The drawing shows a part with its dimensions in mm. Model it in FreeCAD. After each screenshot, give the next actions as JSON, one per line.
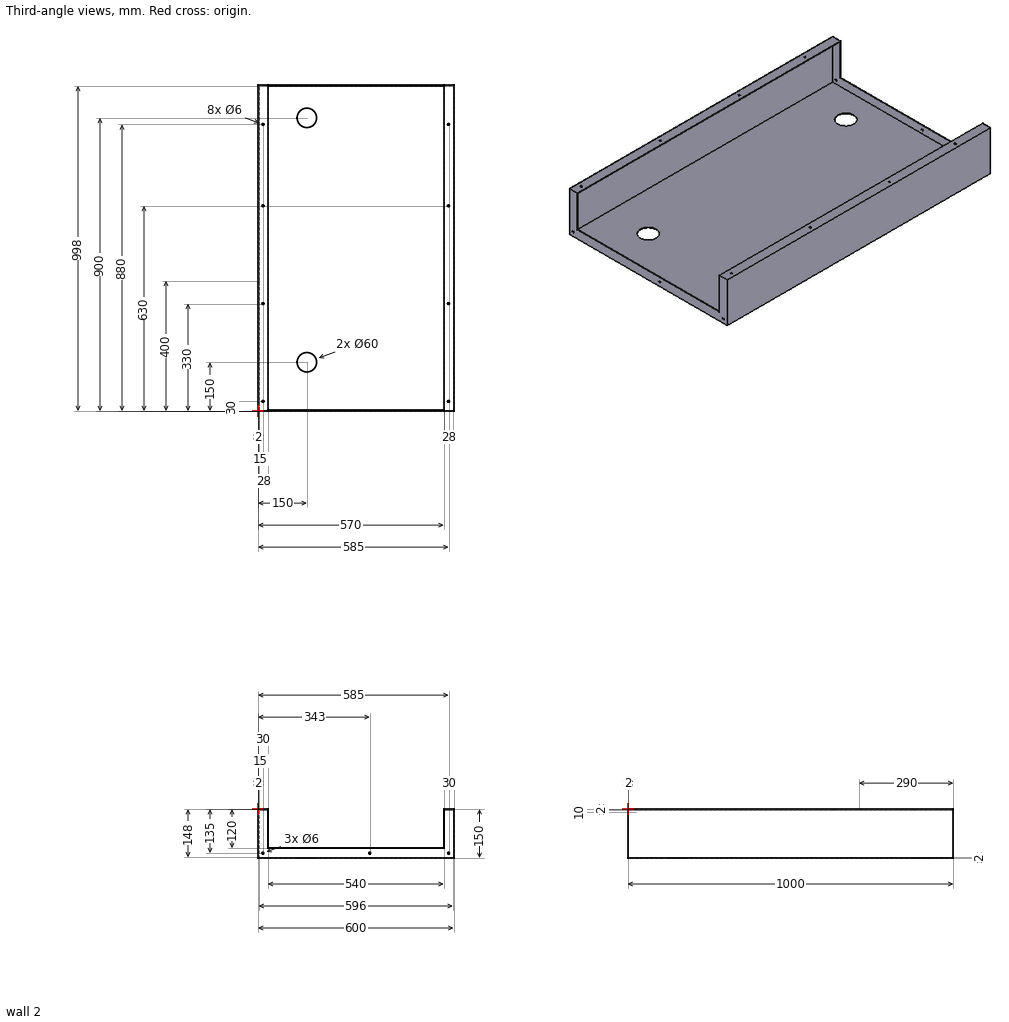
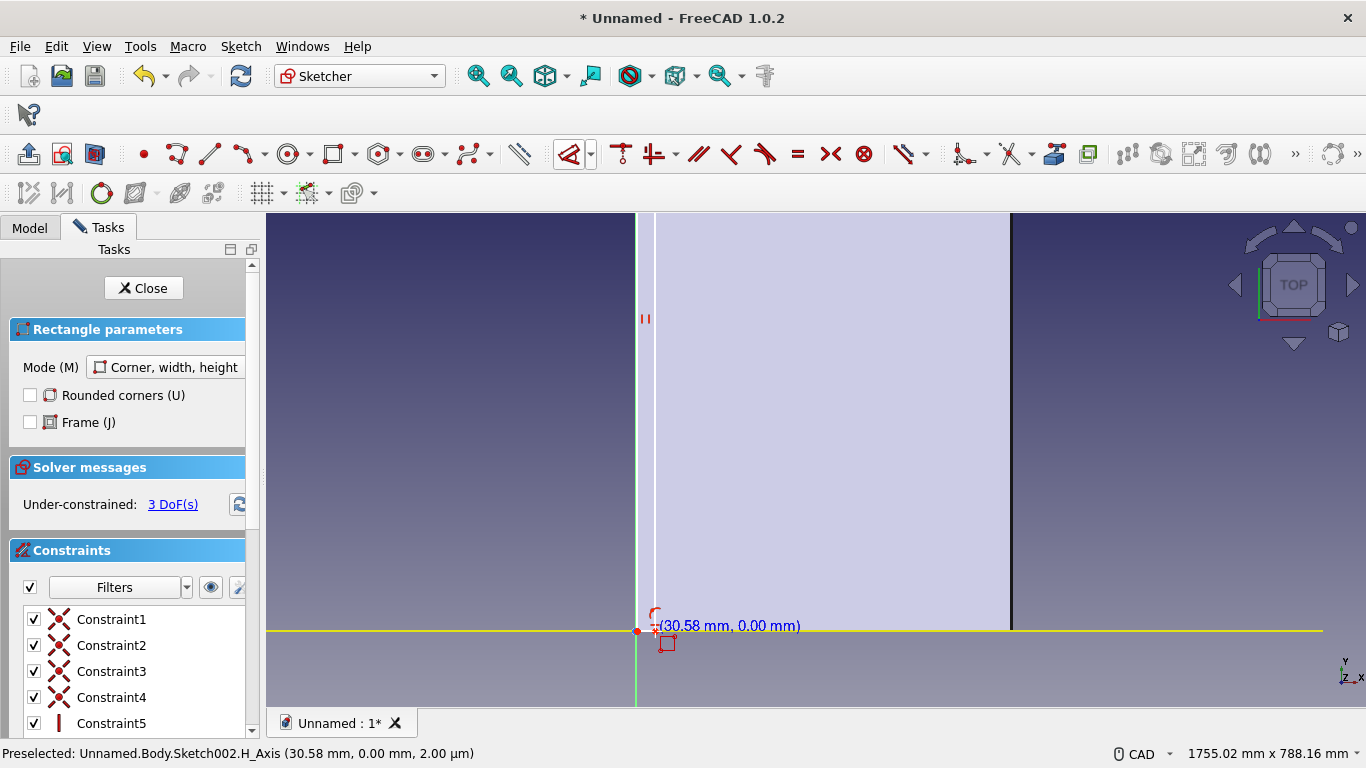
{"action": "scroll", "coordinate": [686, 575], "scroll_direction": "down", "scroll_amount": 4}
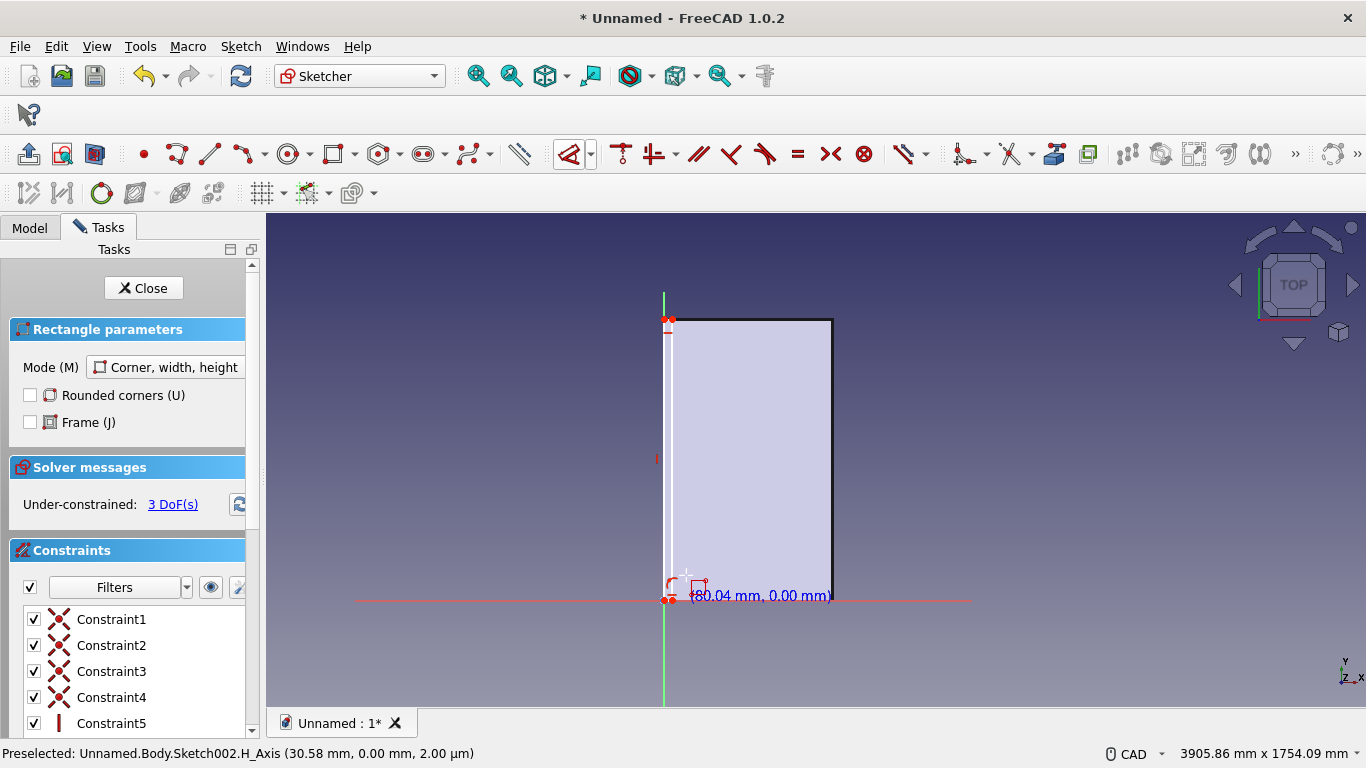
{"action": "scroll", "coordinate": [824, 320], "scroll_direction": "up", "scroll_amount": 4}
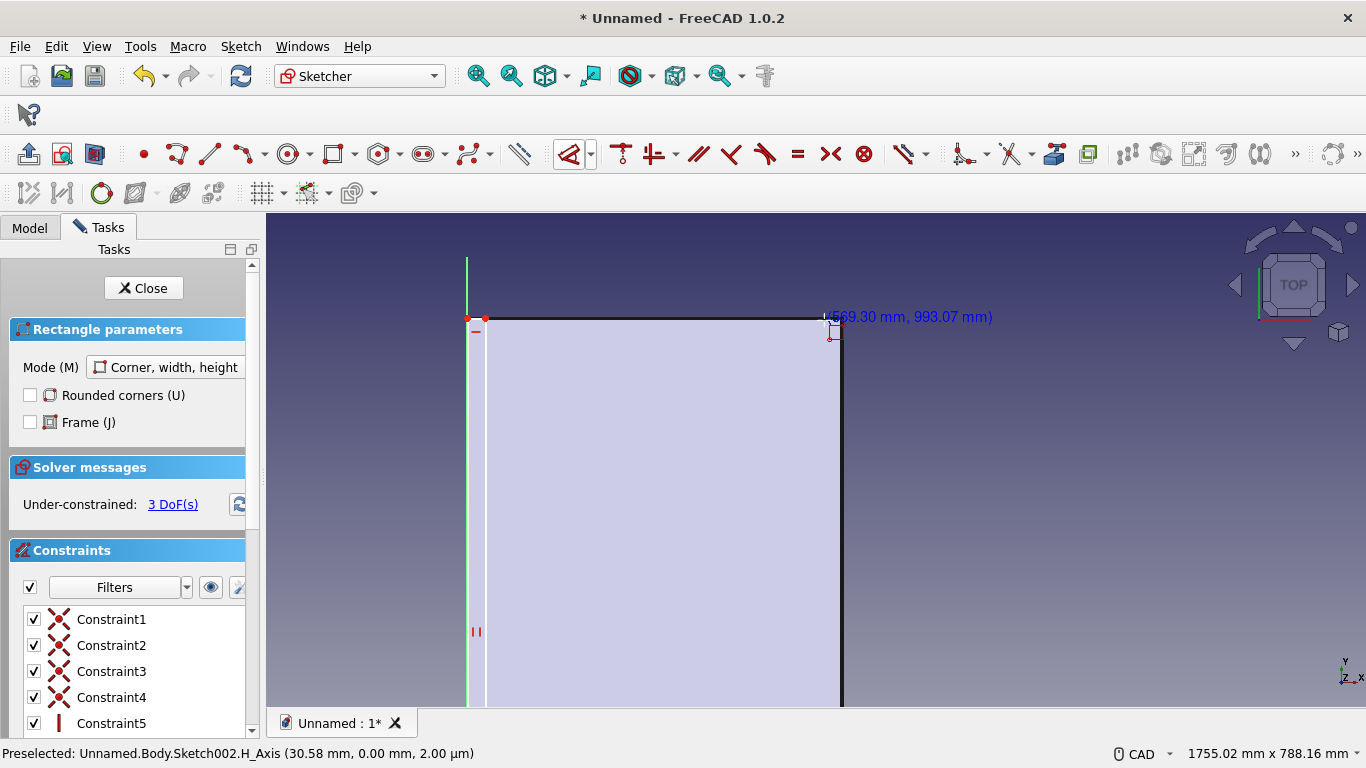
{"action": "left_click", "coordinate": [824, 319]}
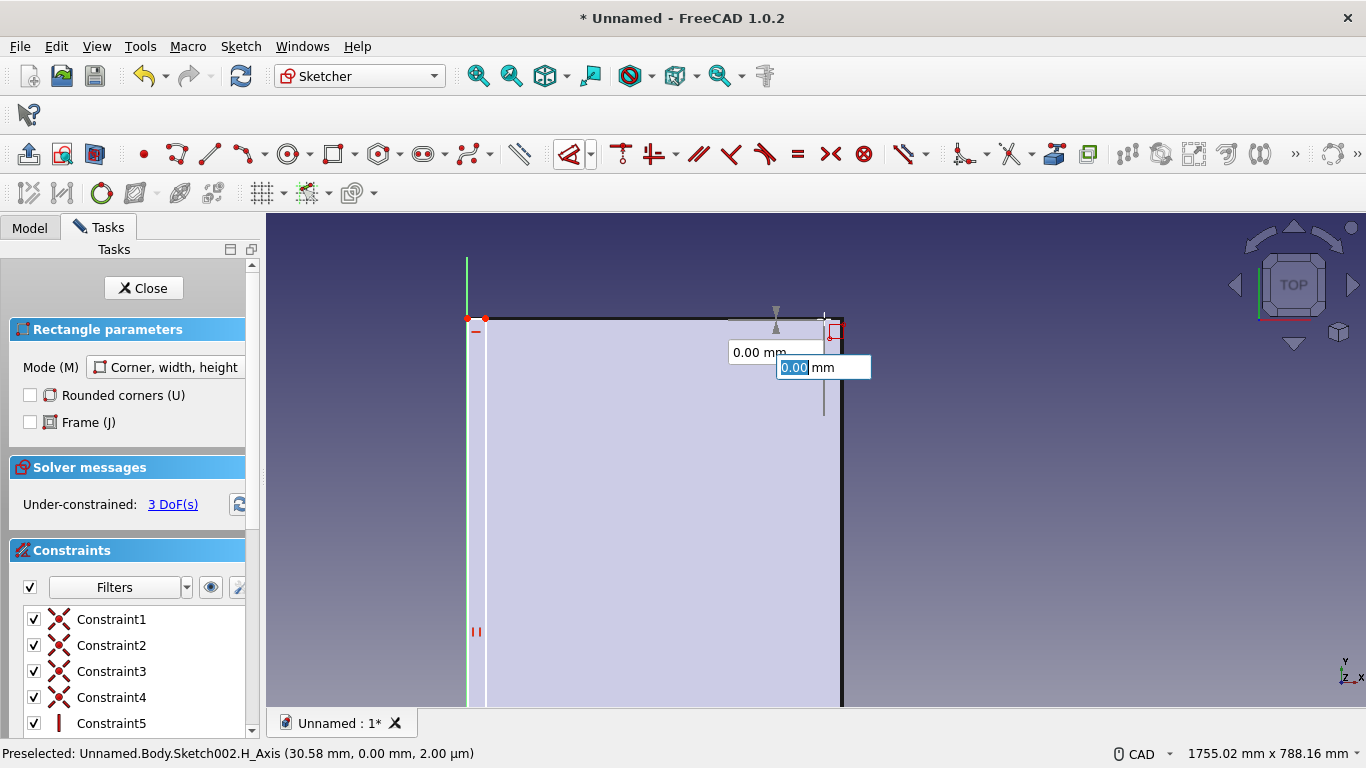
{"action": "scroll", "coordinate": [824, 320], "scroll_direction": "down", "scroll_amount": 4}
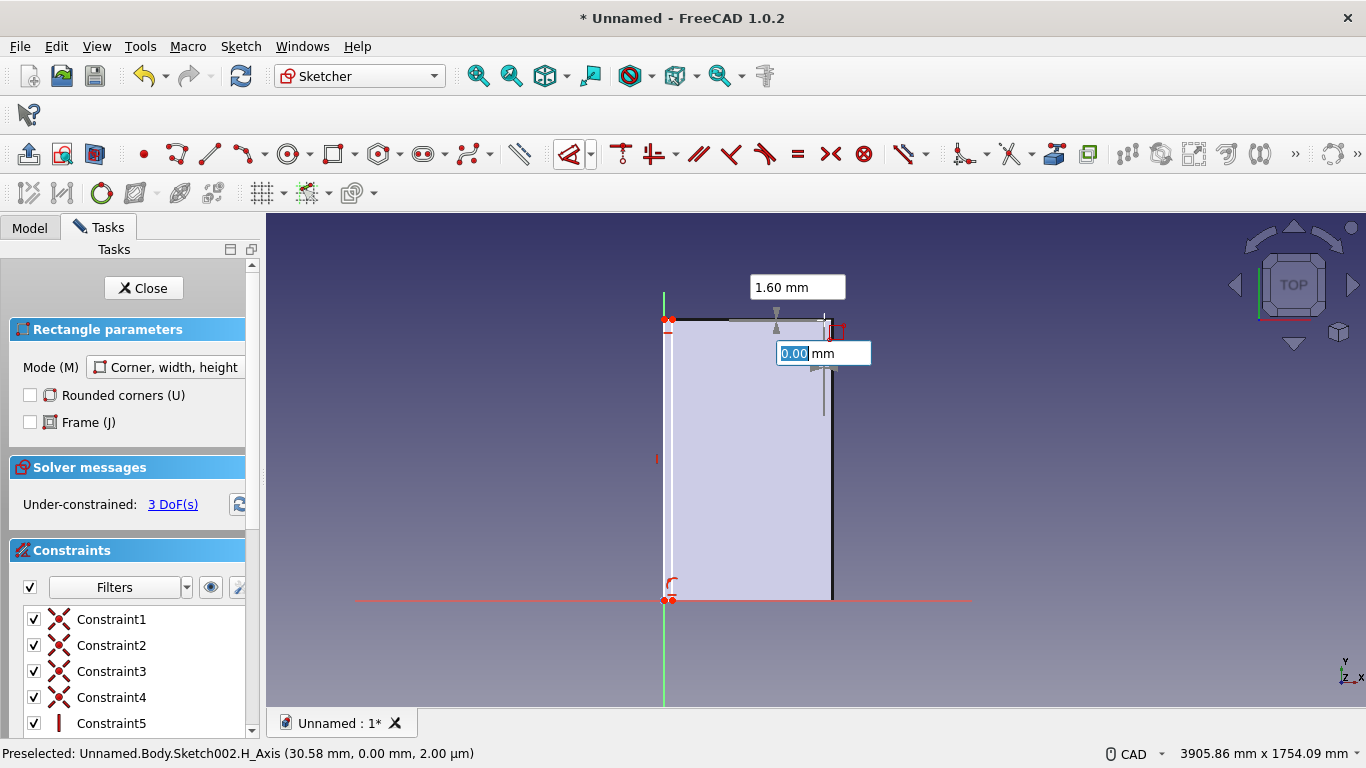
{"action": "left_click", "coordinate": [832, 601]}
{"action": "key", "text": "Escape"}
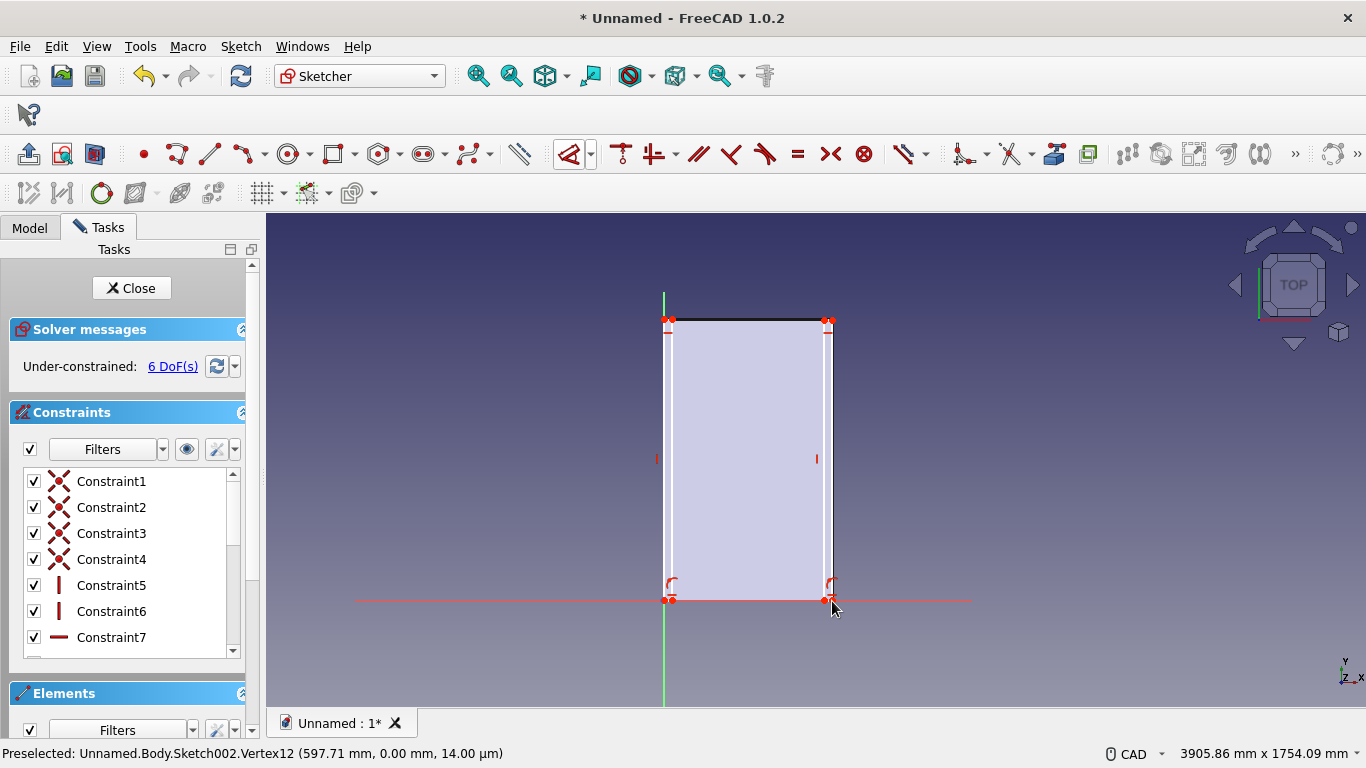
{"action": "scroll", "coordinate": [668, 601], "scroll_direction": "up", "scroll_amount": 9}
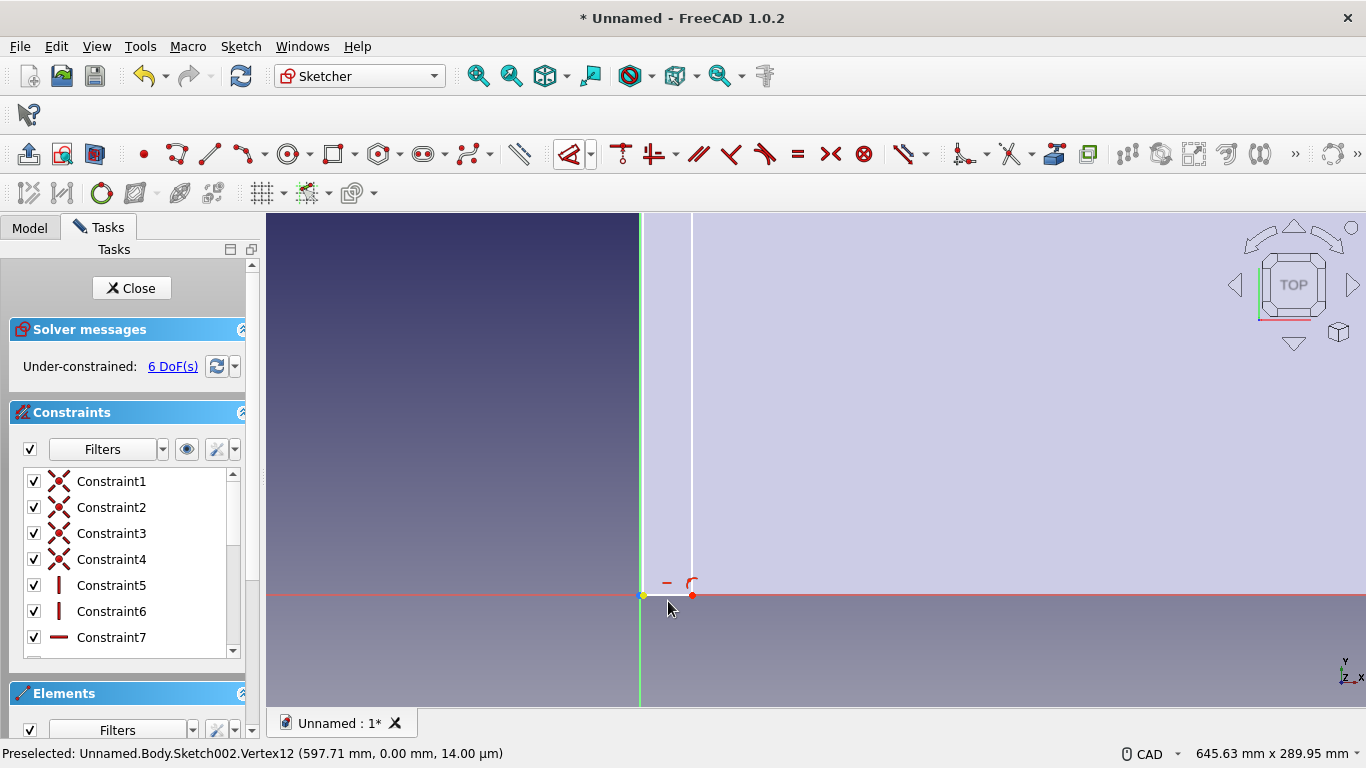
{"action": "left_click", "coordinate": [668, 595]}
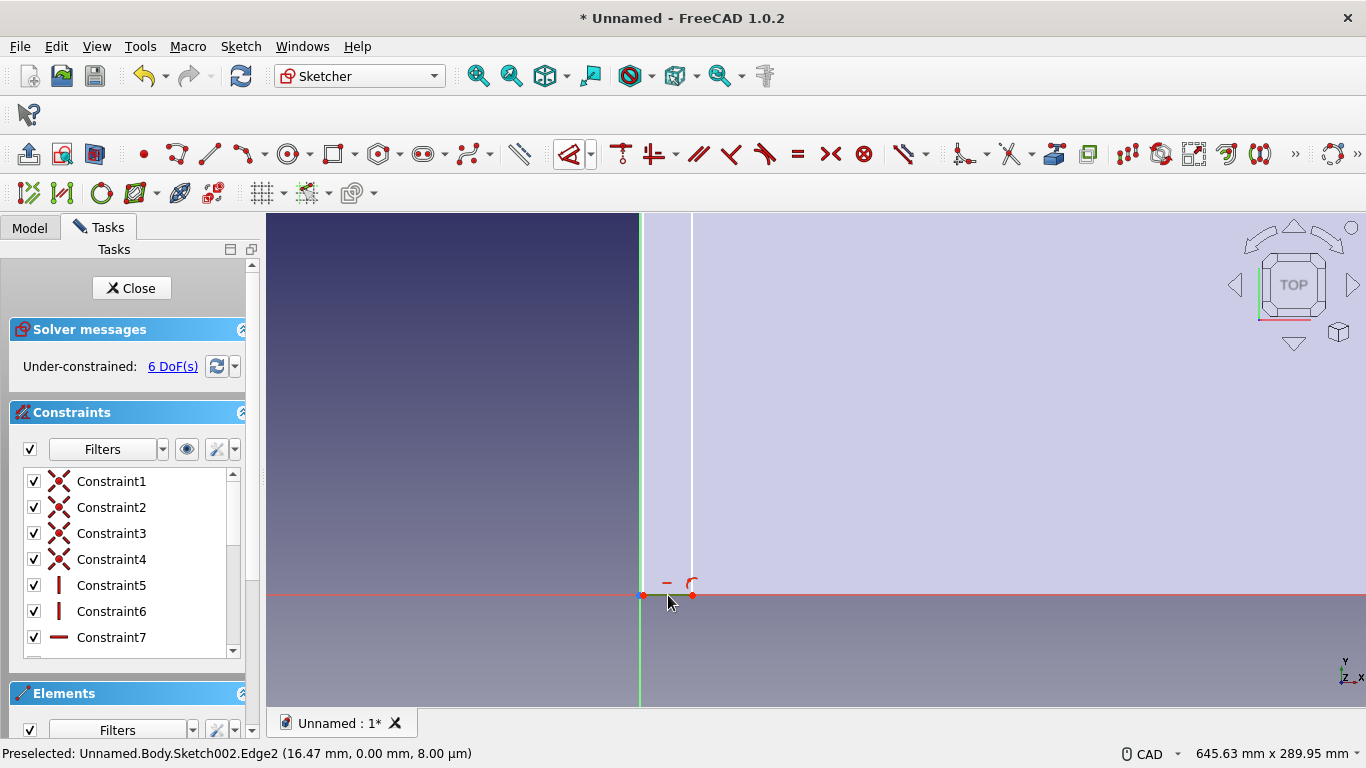
{"action": "left_click", "coordinate": [590, 154]}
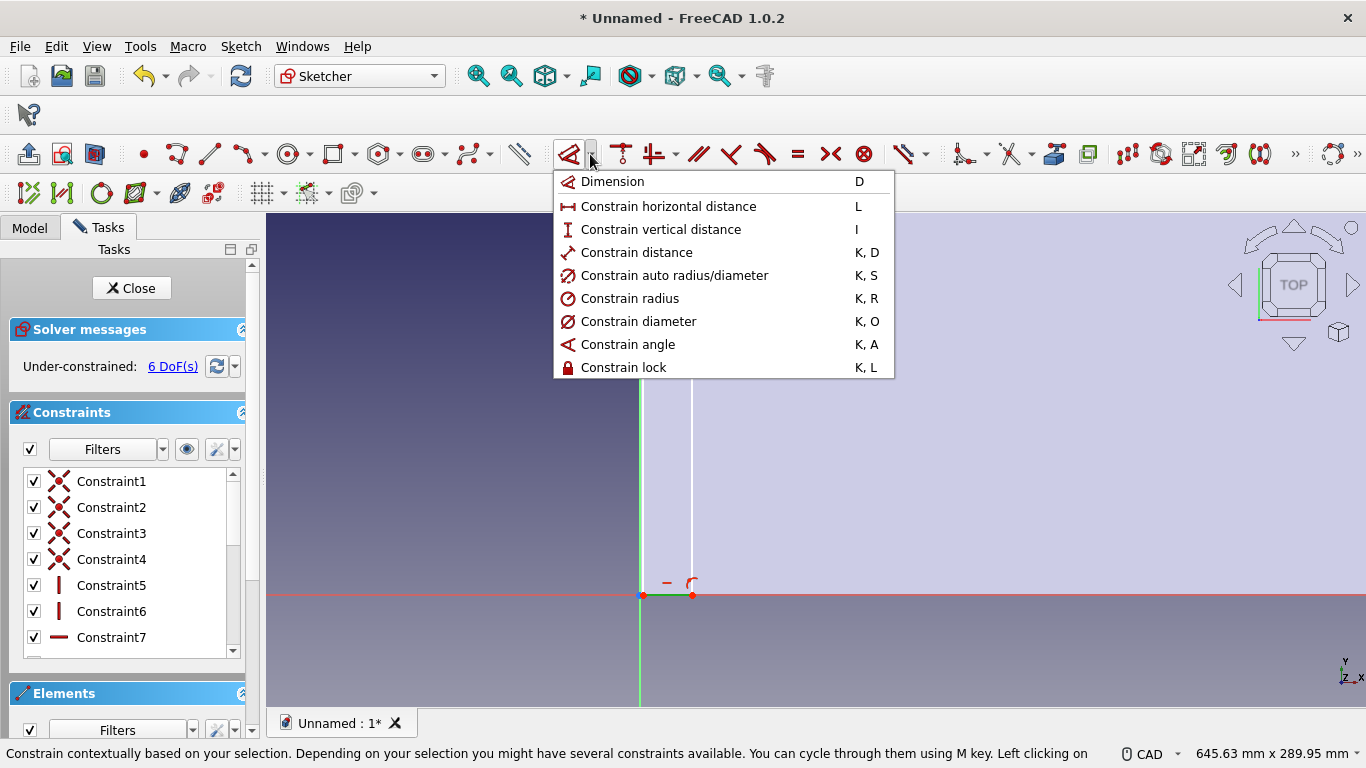
{"action": "left_click", "coordinate": [724, 206]}